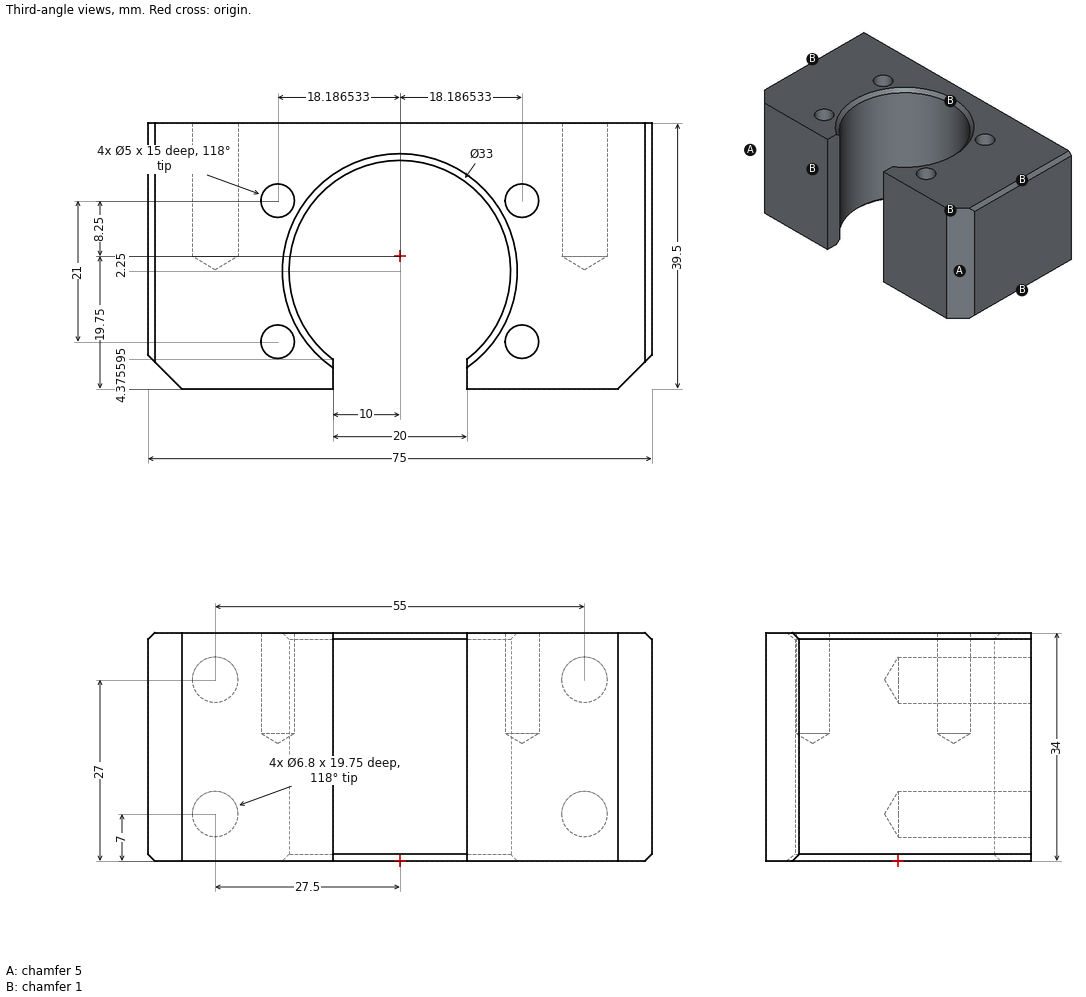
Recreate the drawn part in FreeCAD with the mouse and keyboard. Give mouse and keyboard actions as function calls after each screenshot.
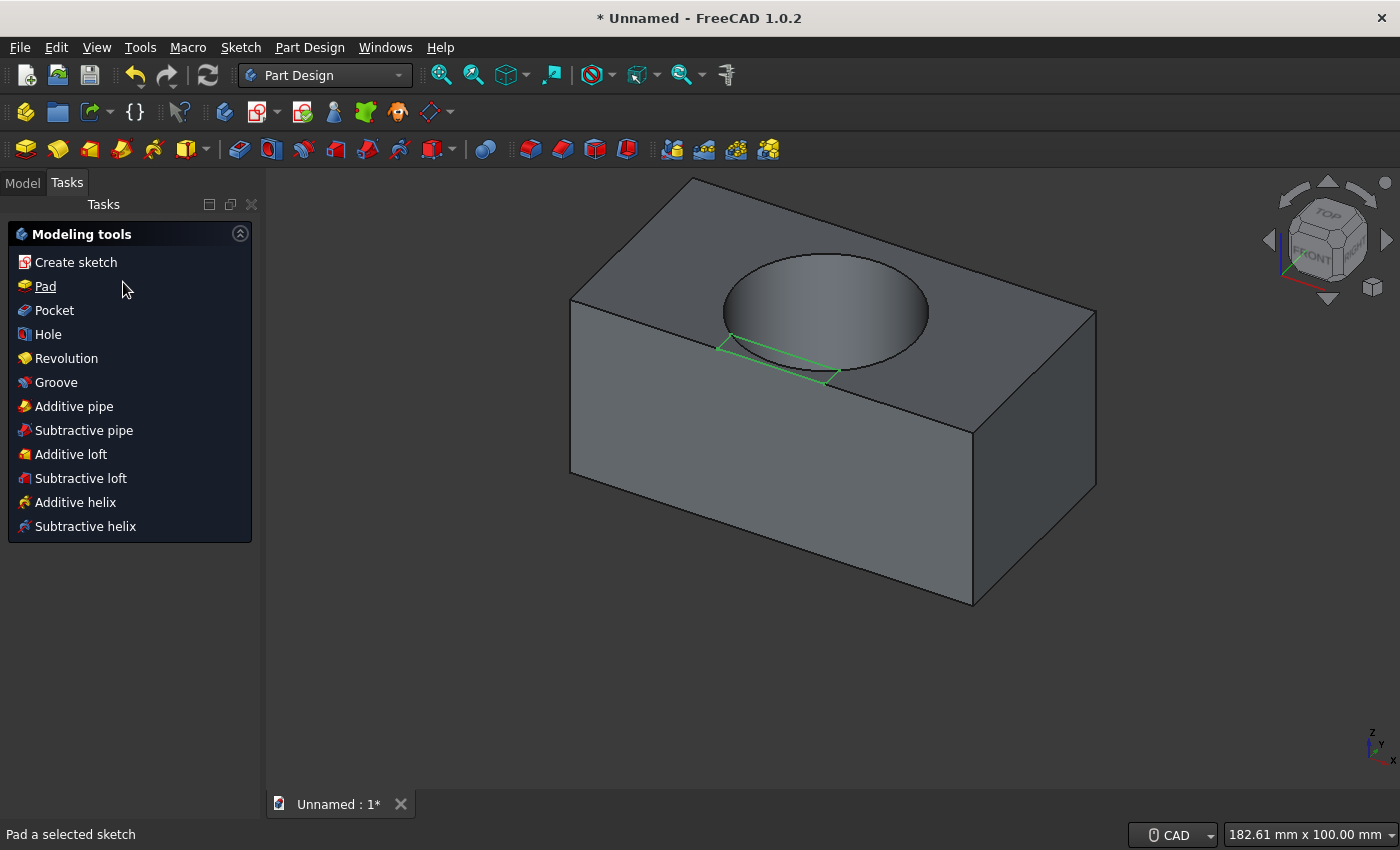
click(240, 150)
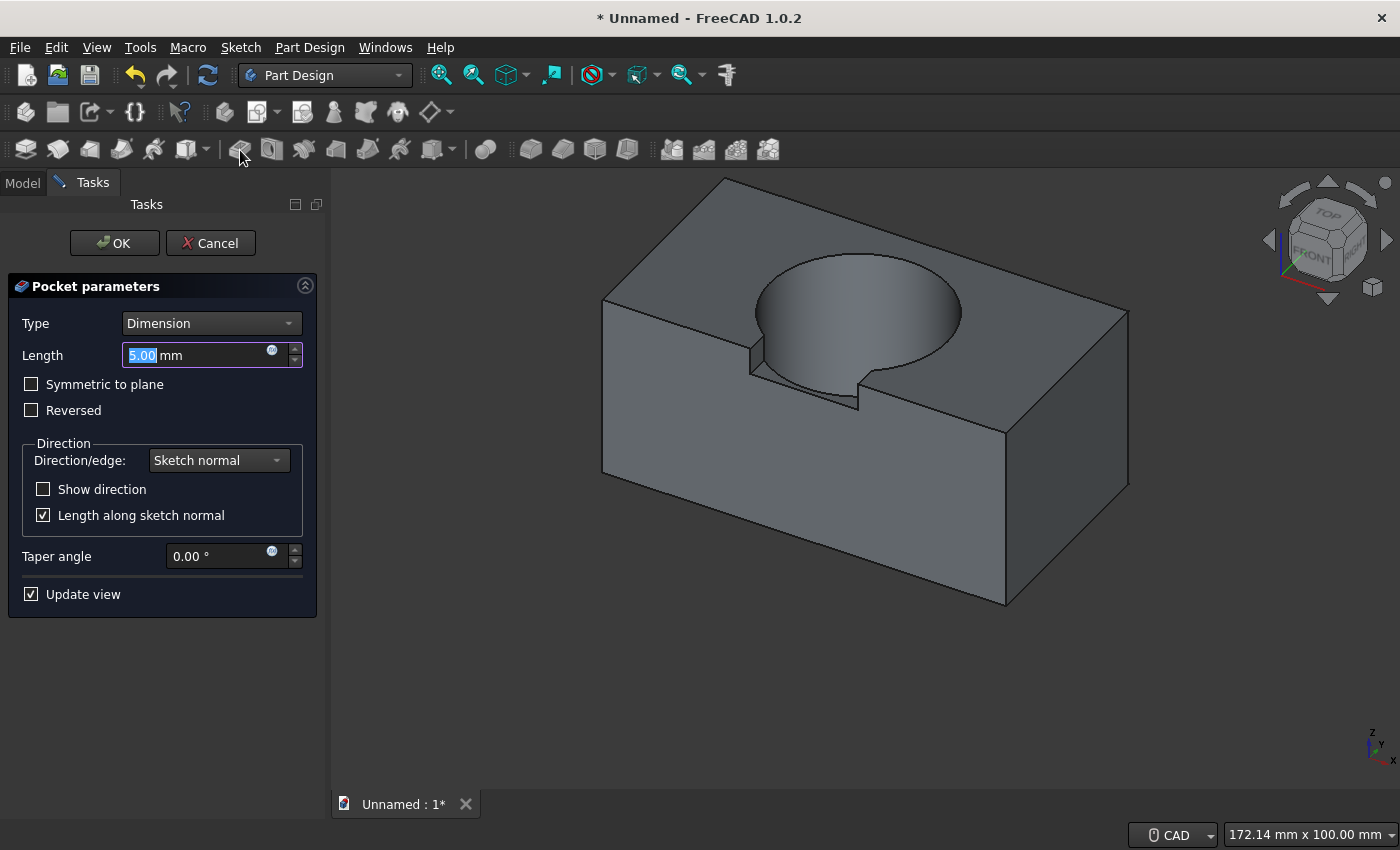
click(212, 324)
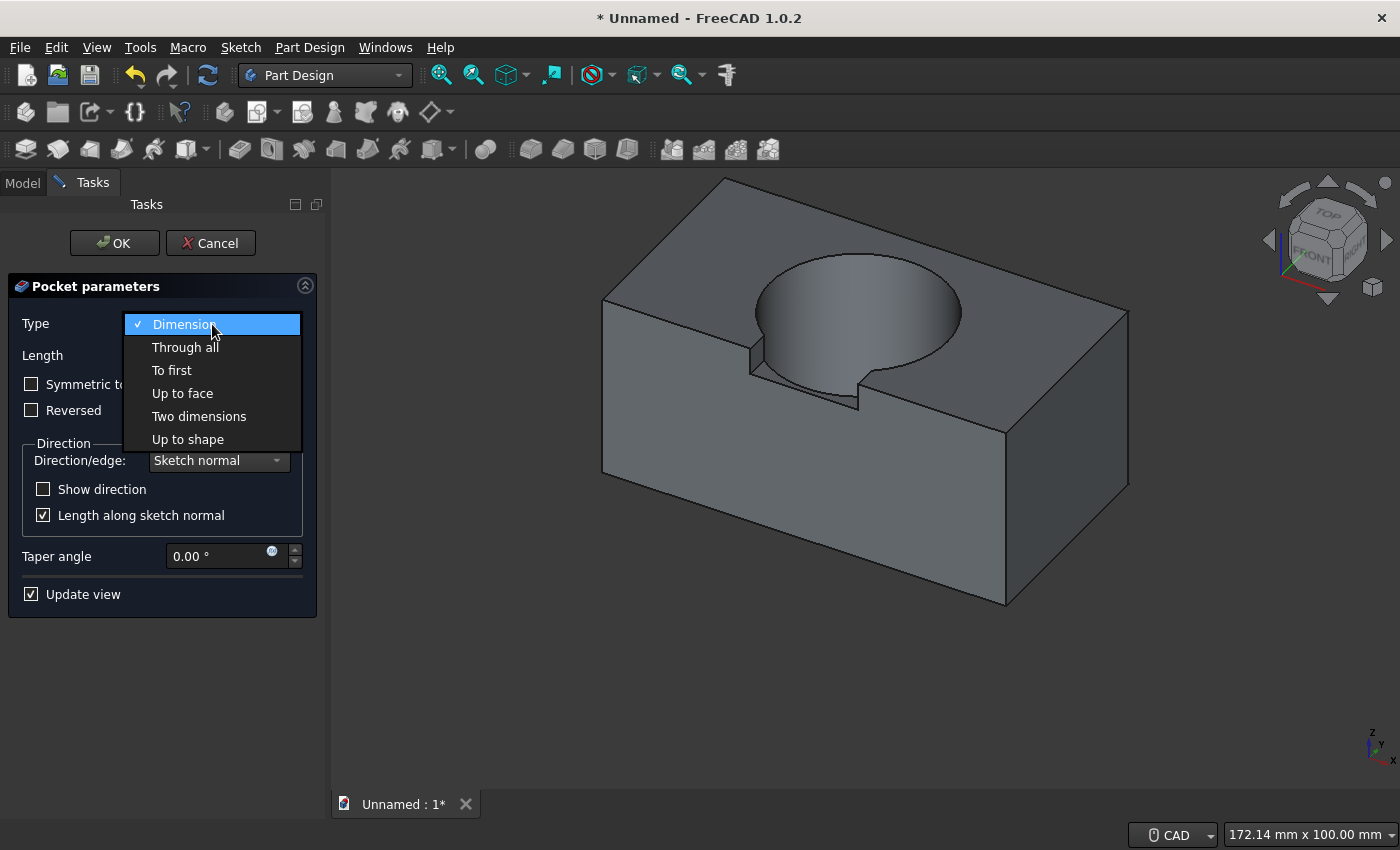
click(212, 348)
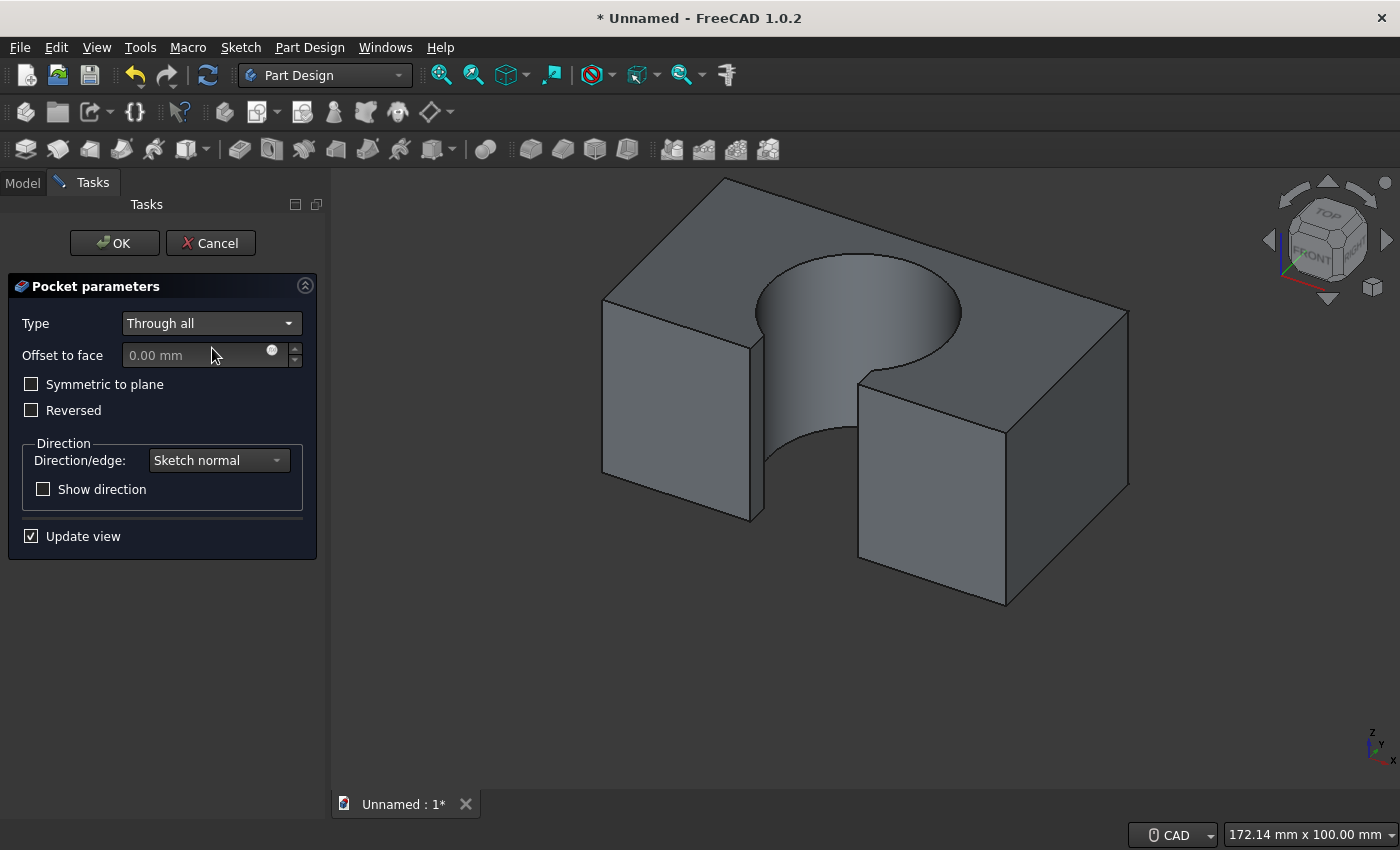
click(115, 243)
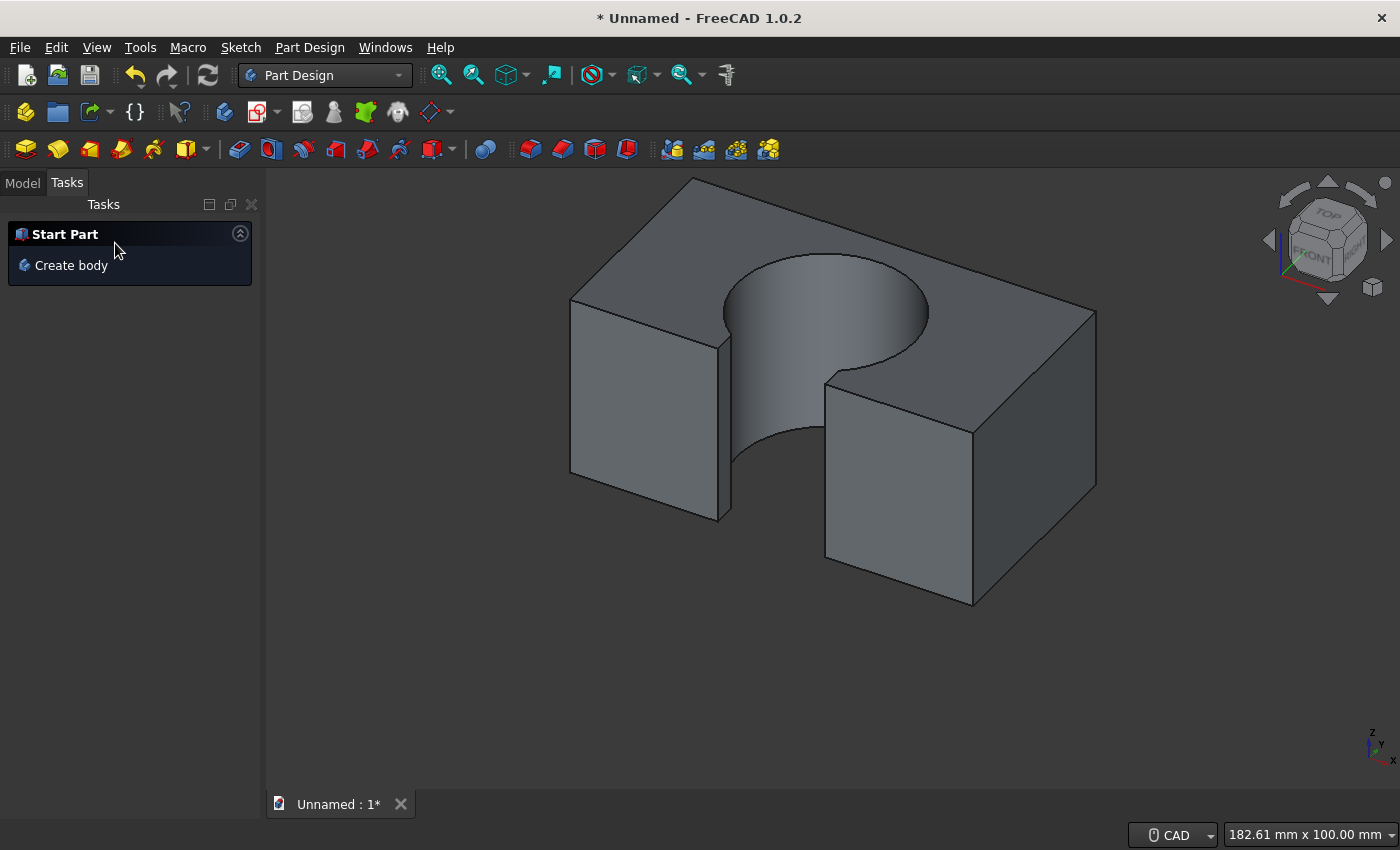
key(4)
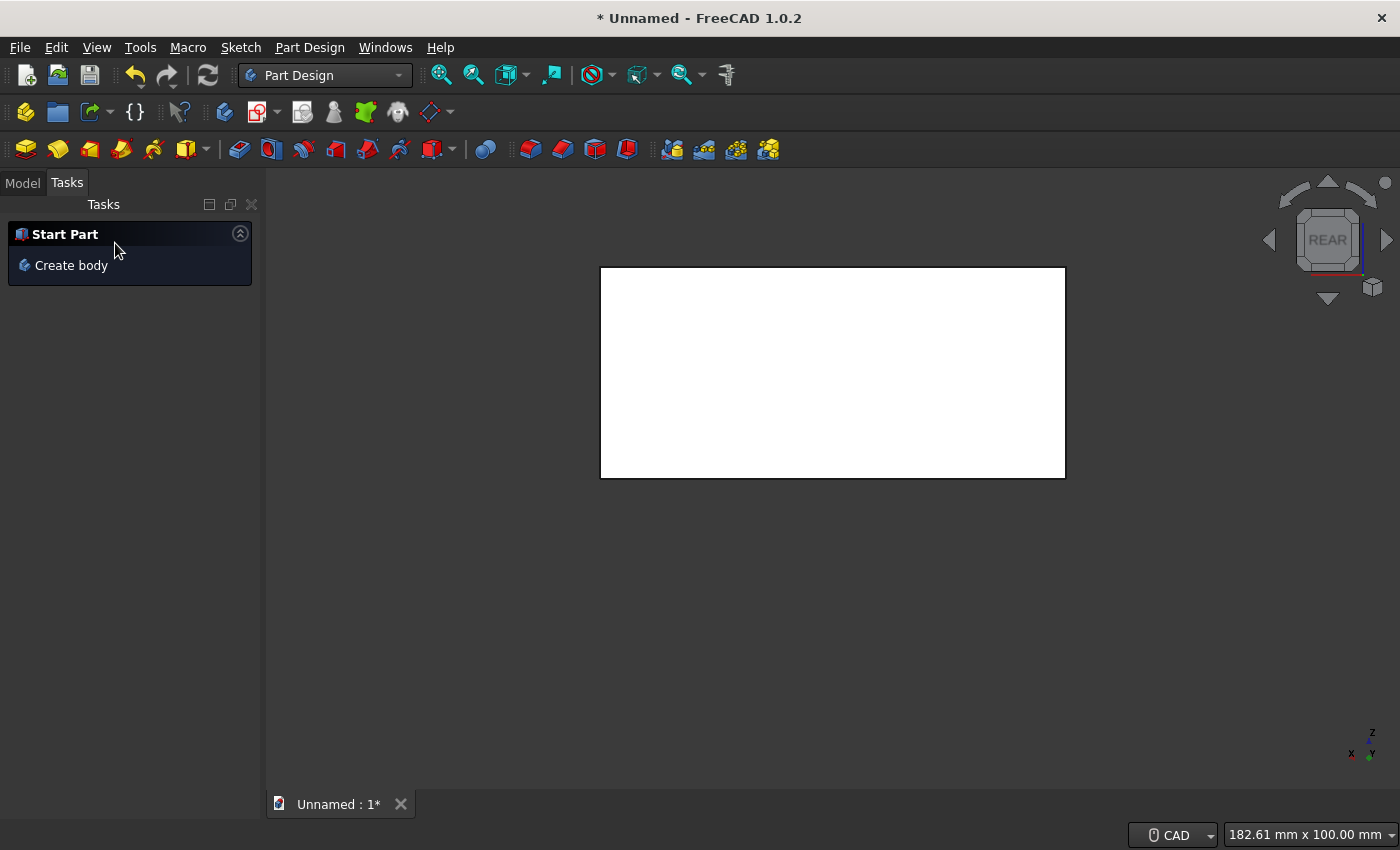
click(442, 76)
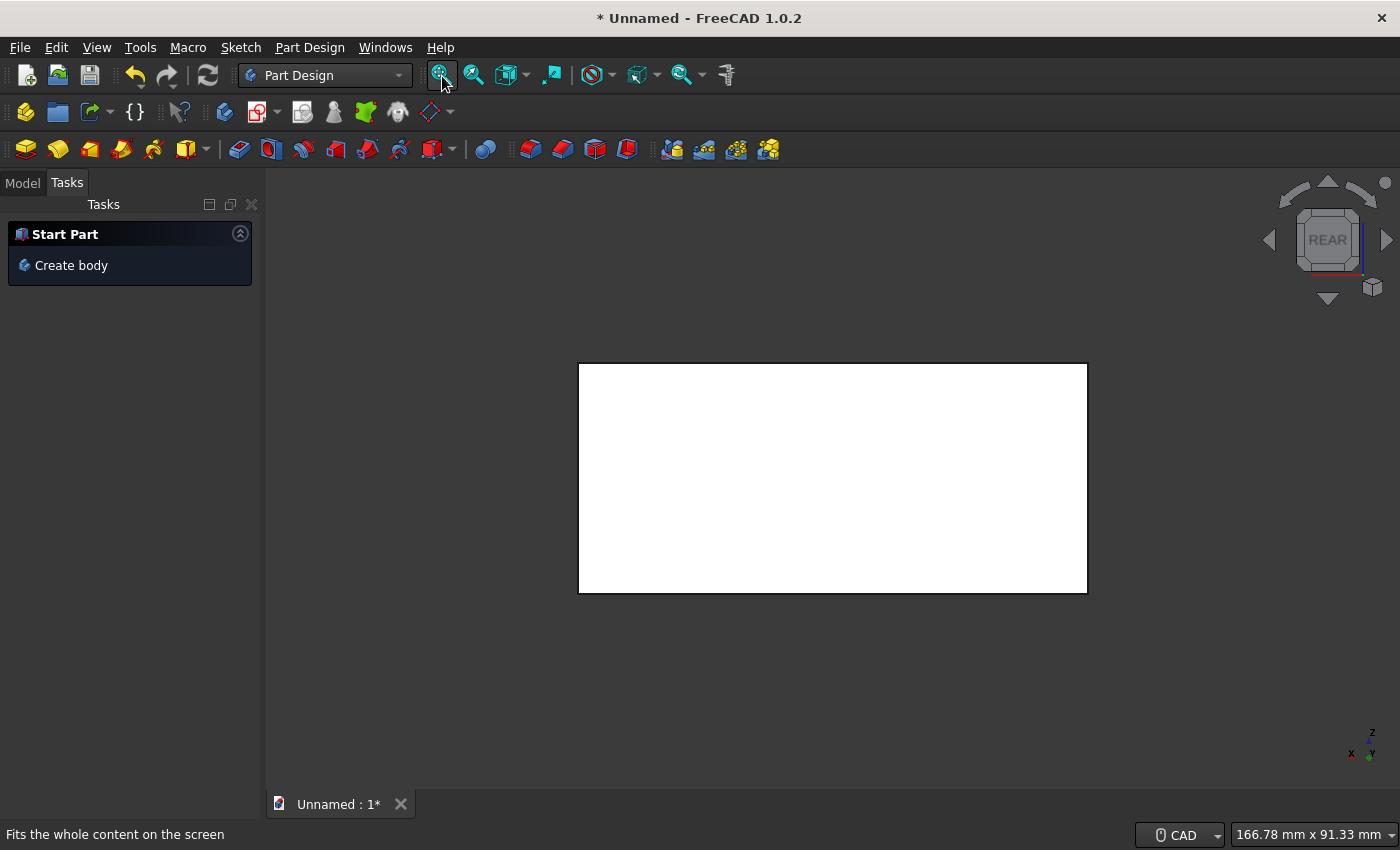
click(760, 478)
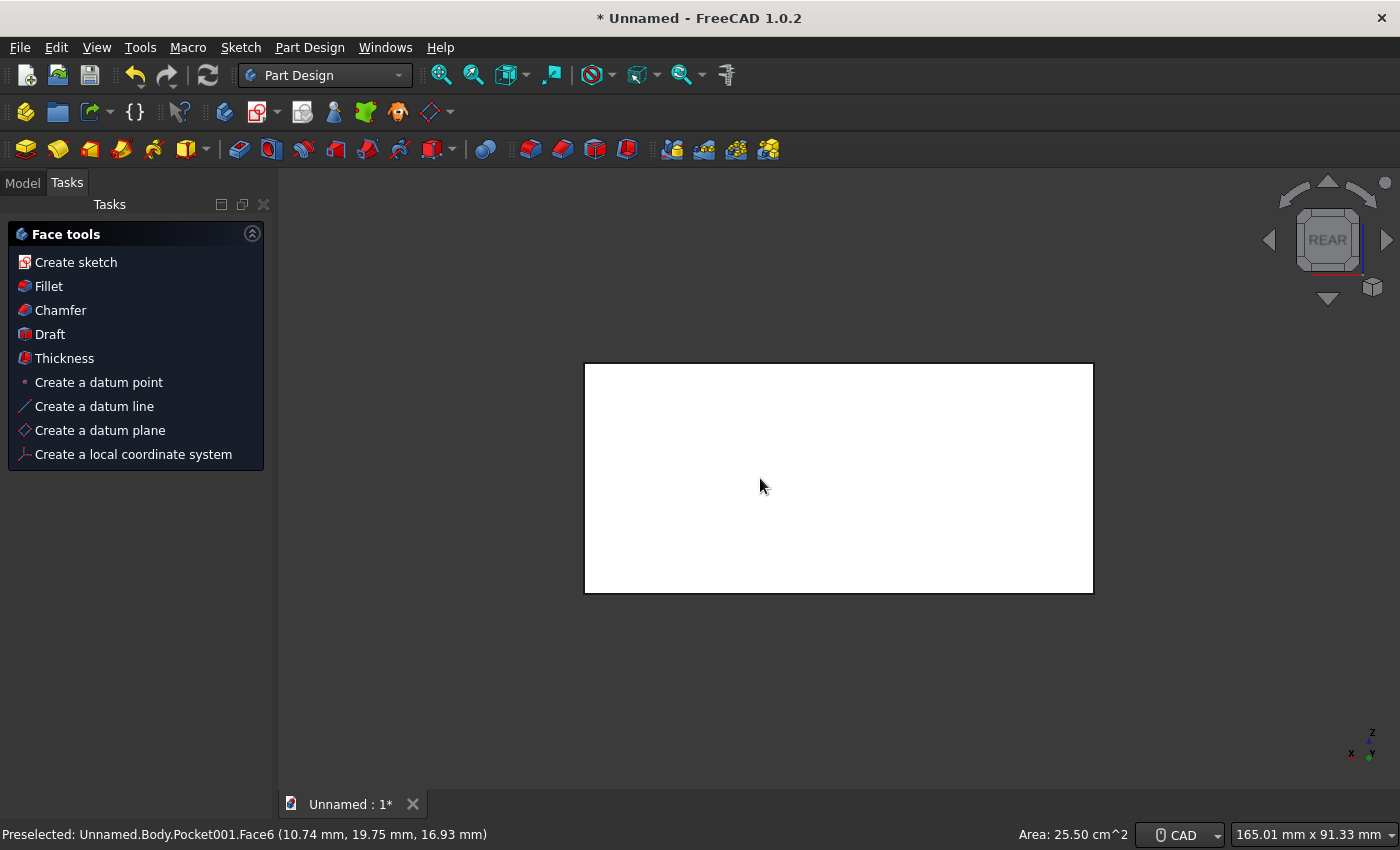
click(258, 112)